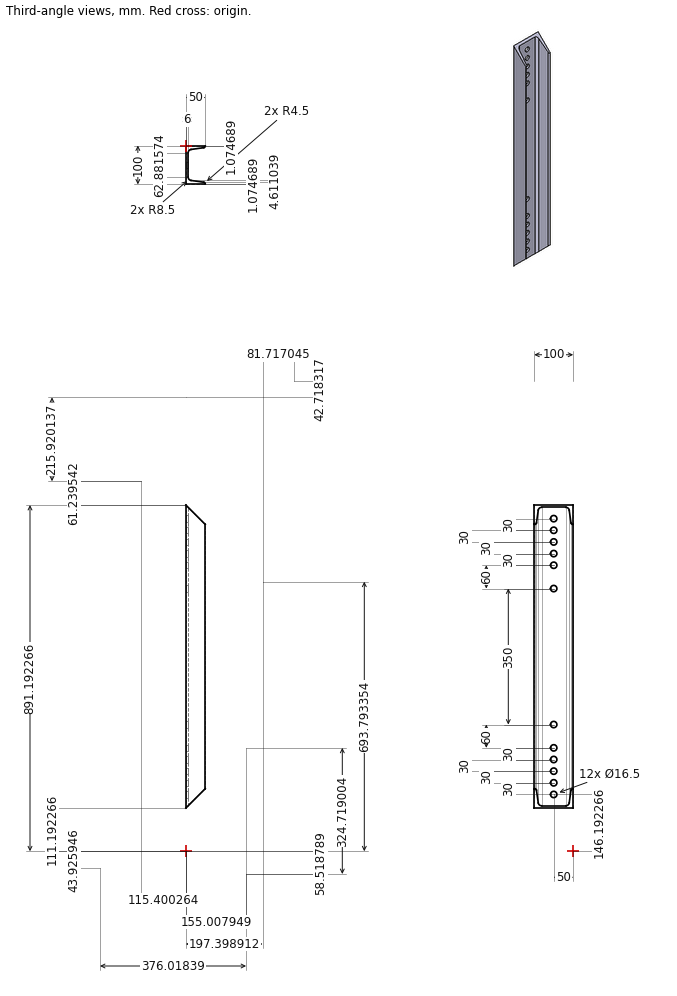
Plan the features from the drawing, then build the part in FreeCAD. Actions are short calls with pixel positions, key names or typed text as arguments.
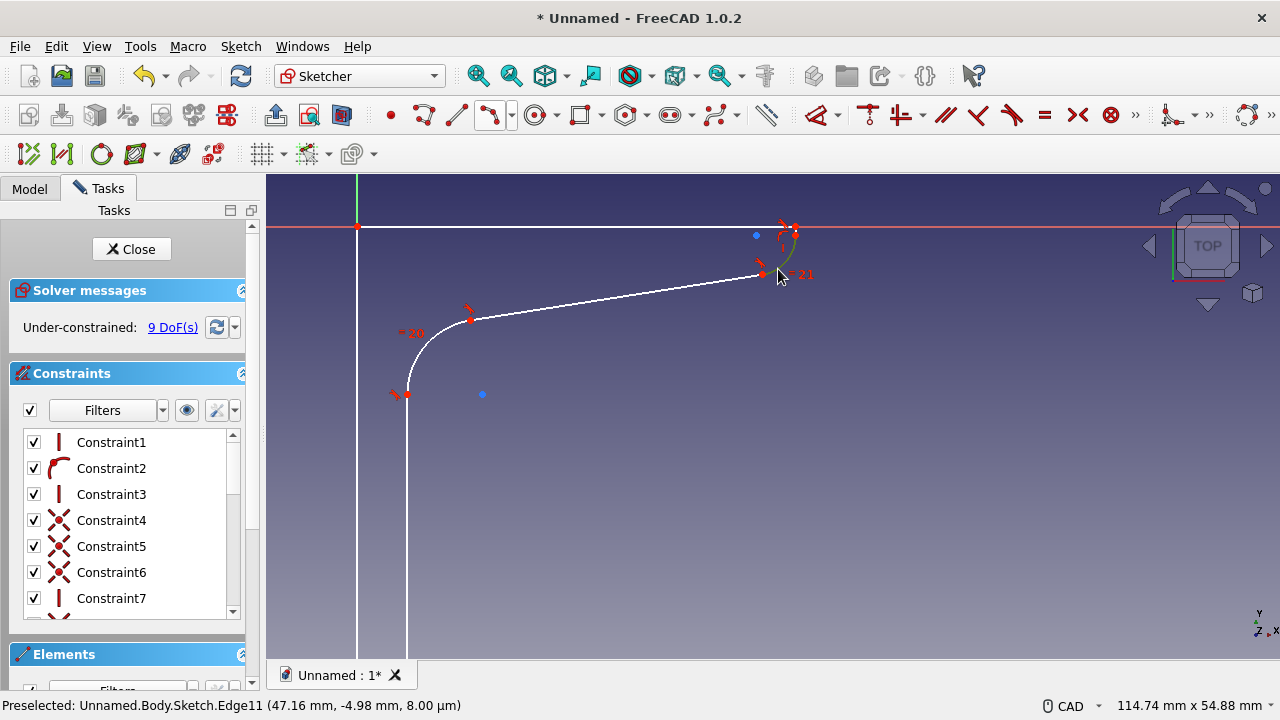
click(838, 116)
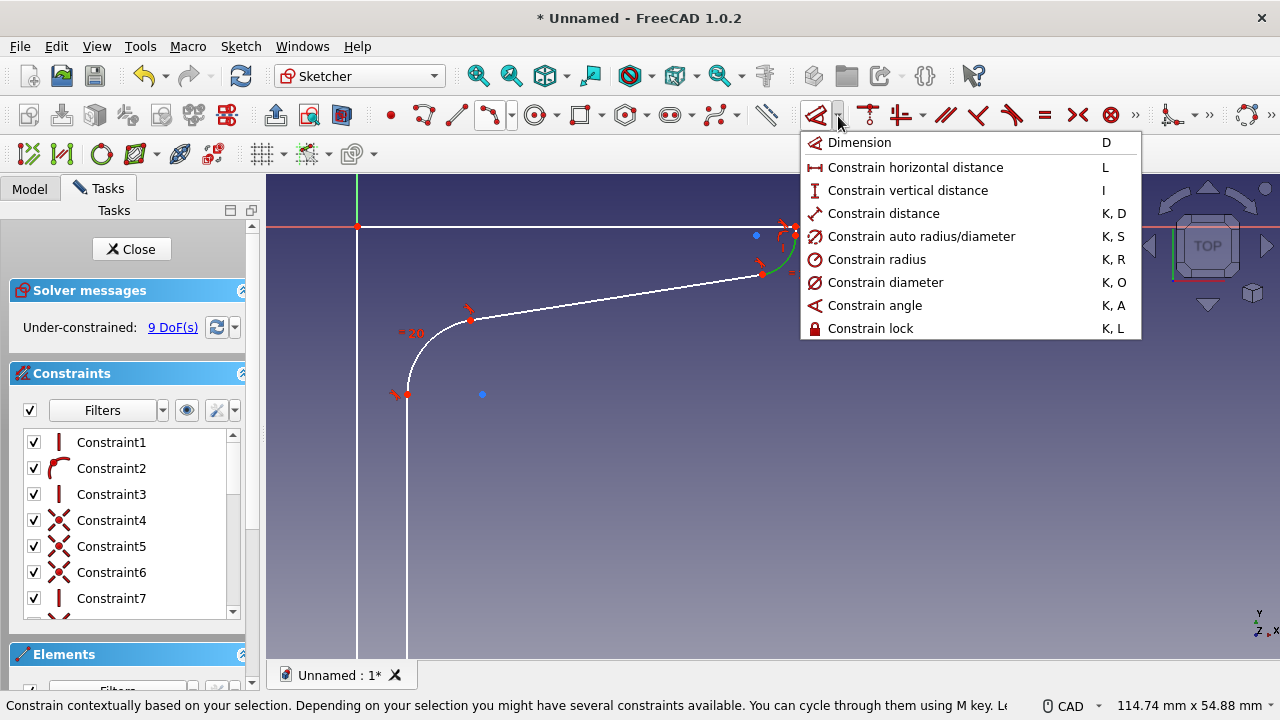
click(971, 260)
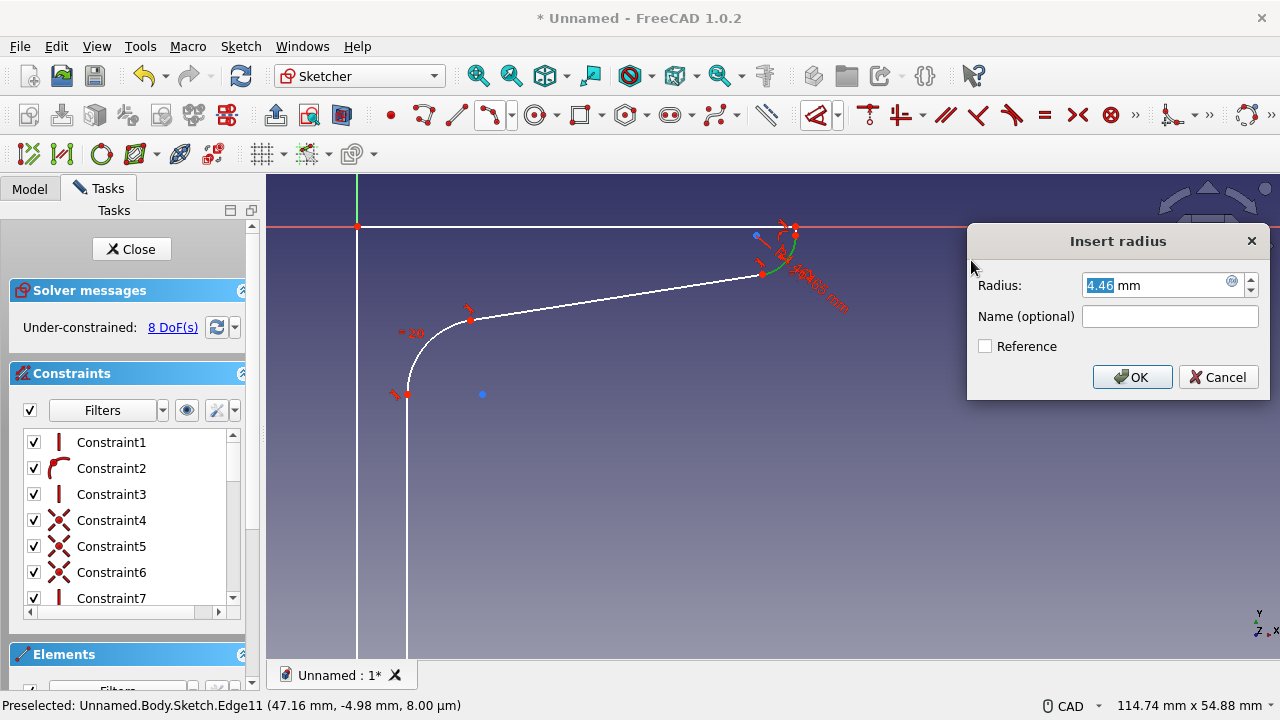
text(4.5)
key(Return)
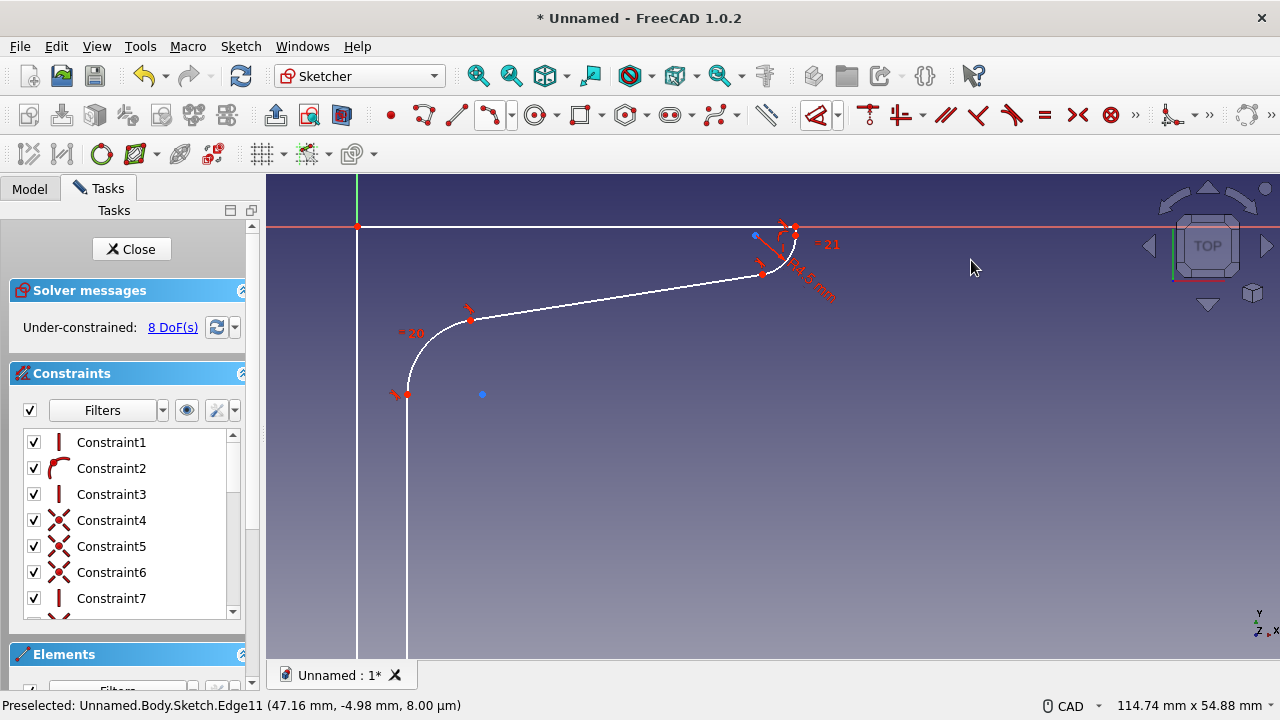
click(664, 227)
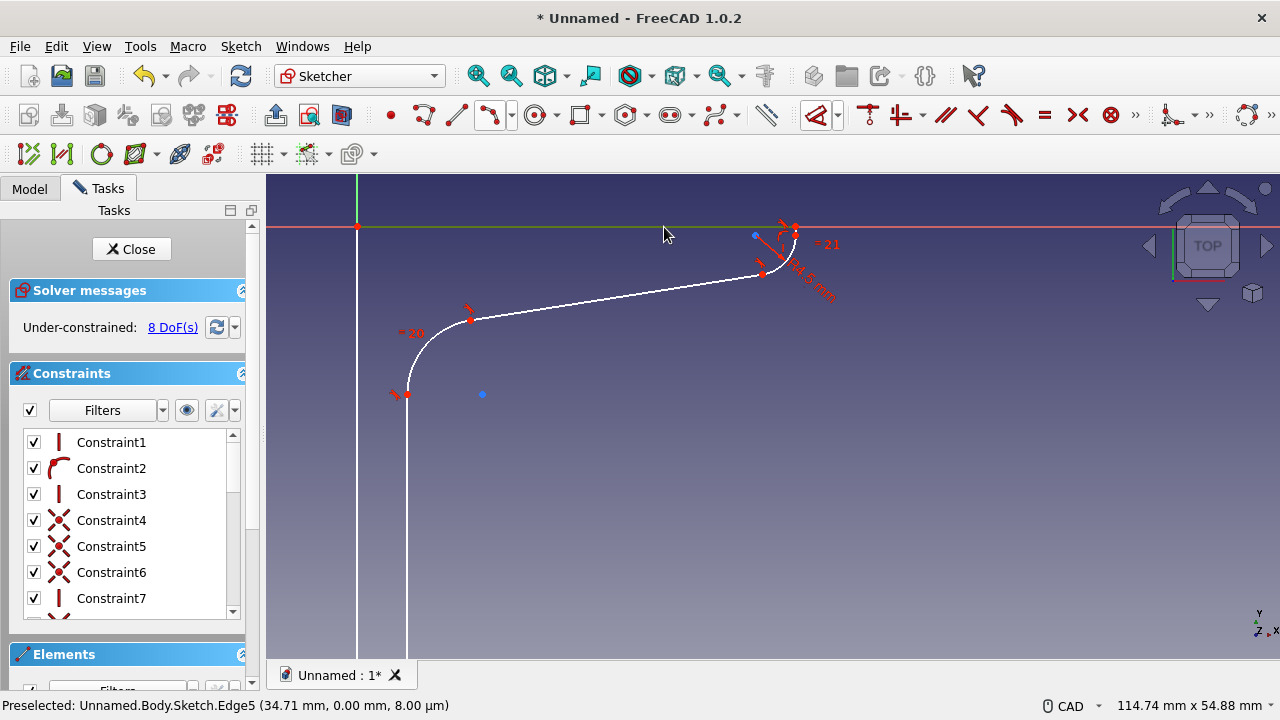
key(l)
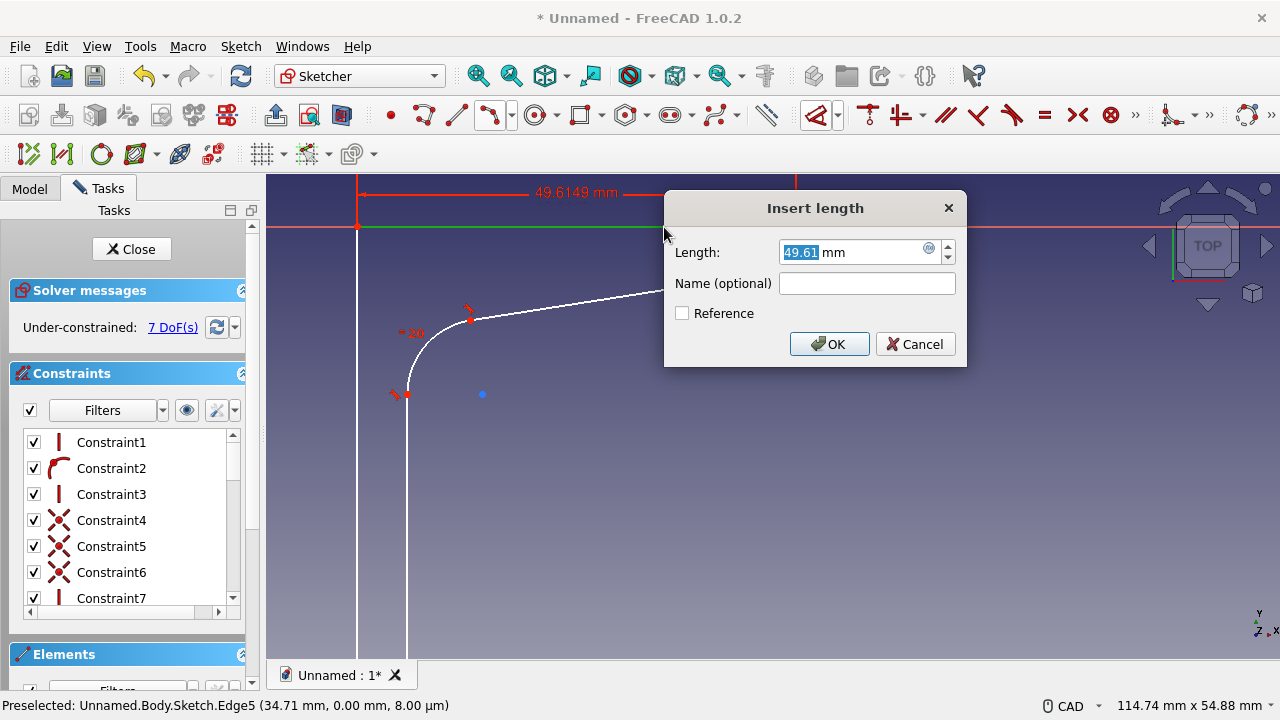
text(50)
key(Return)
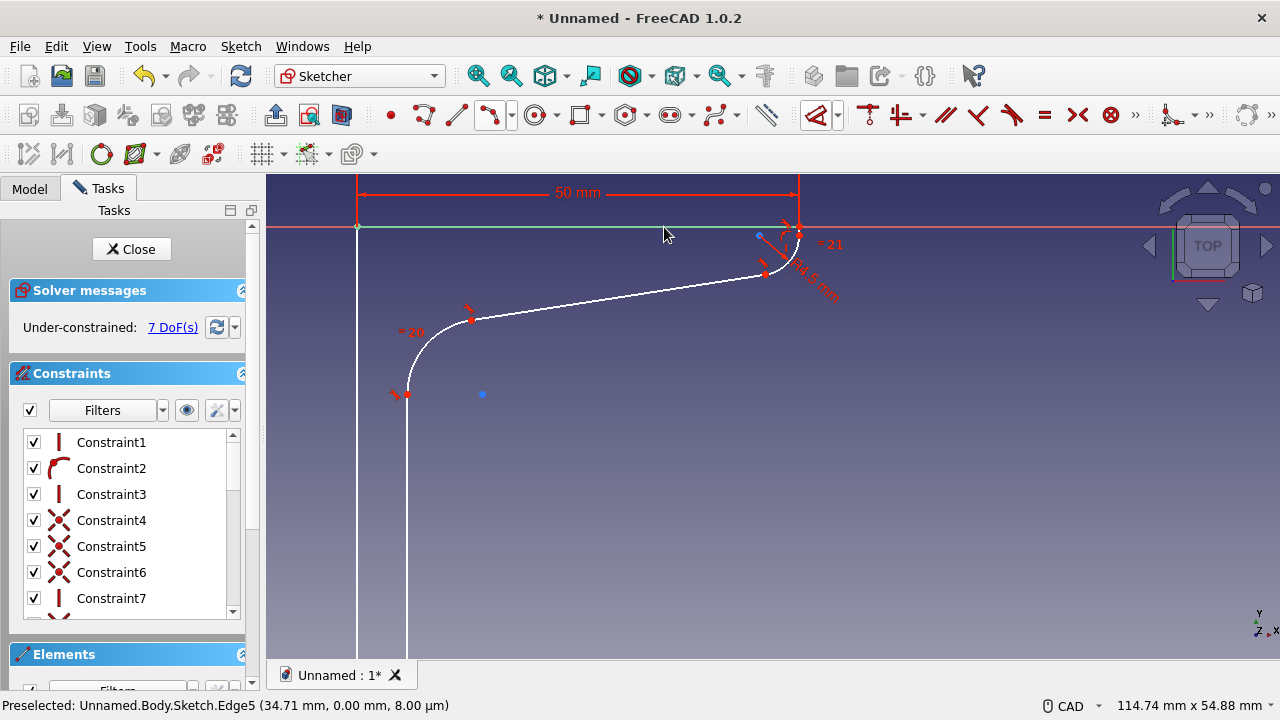
scroll(778, 270, down, 5)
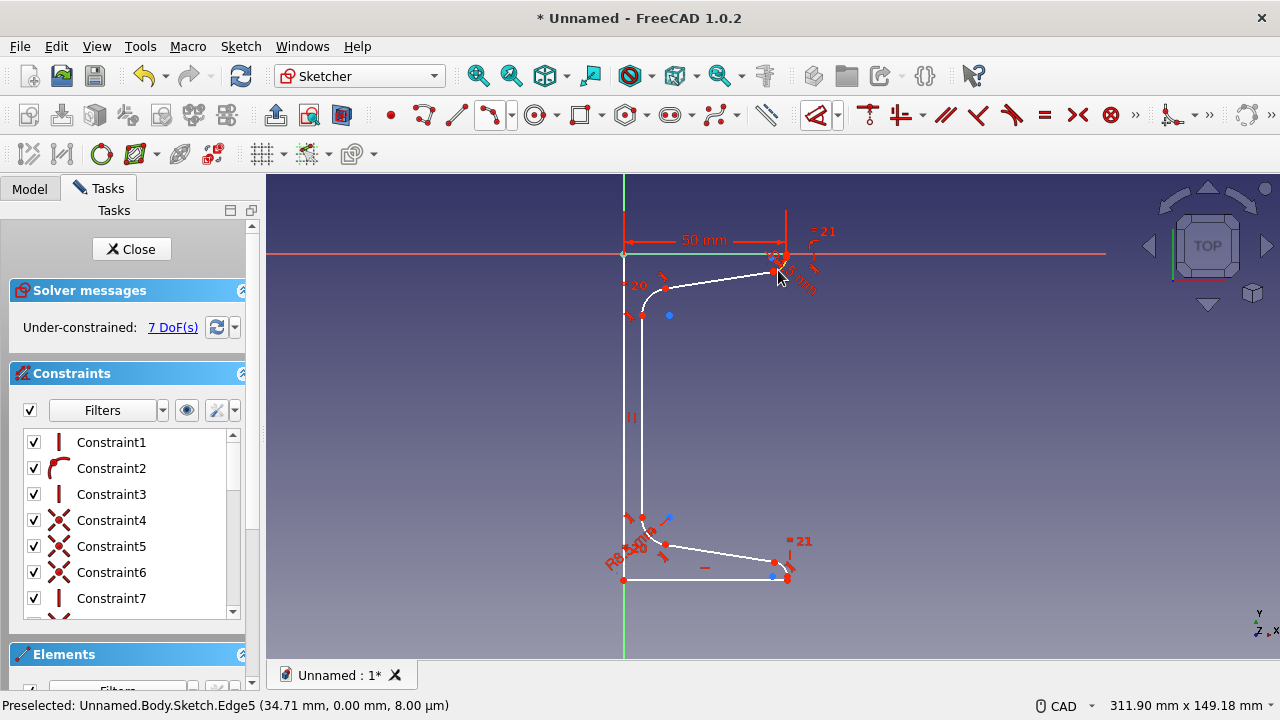
click(673, 580)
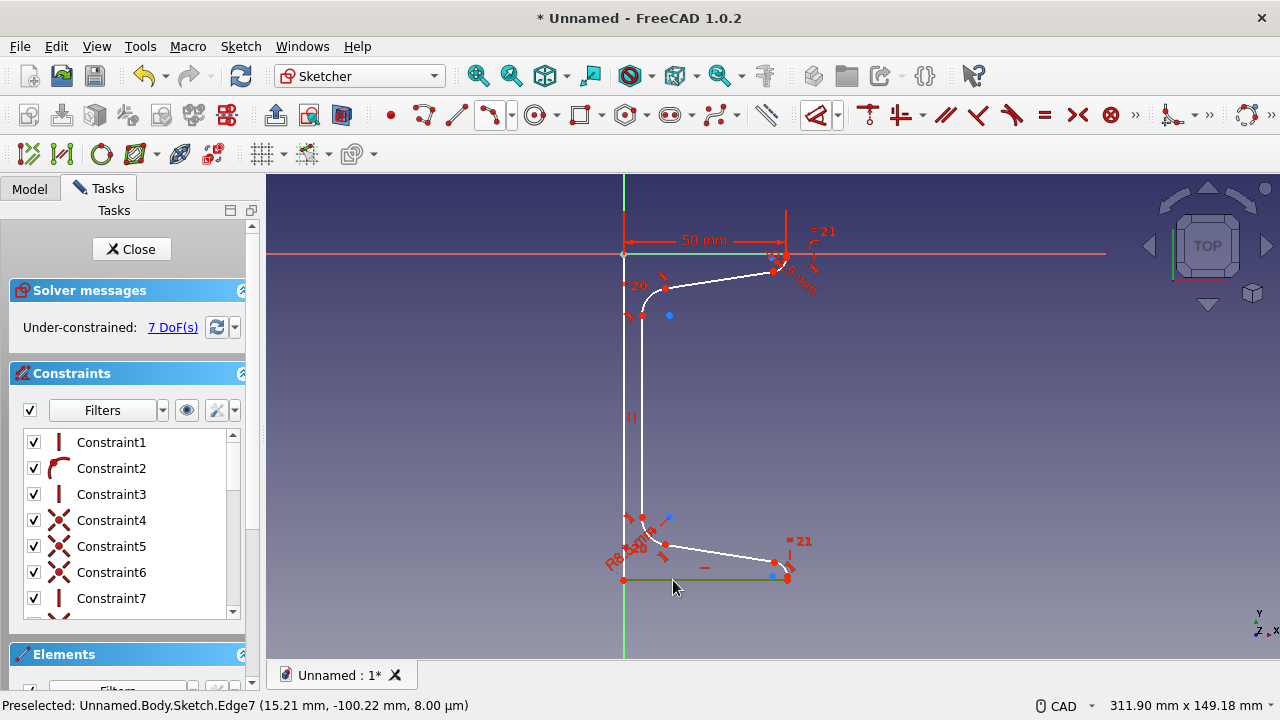
click(838, 116)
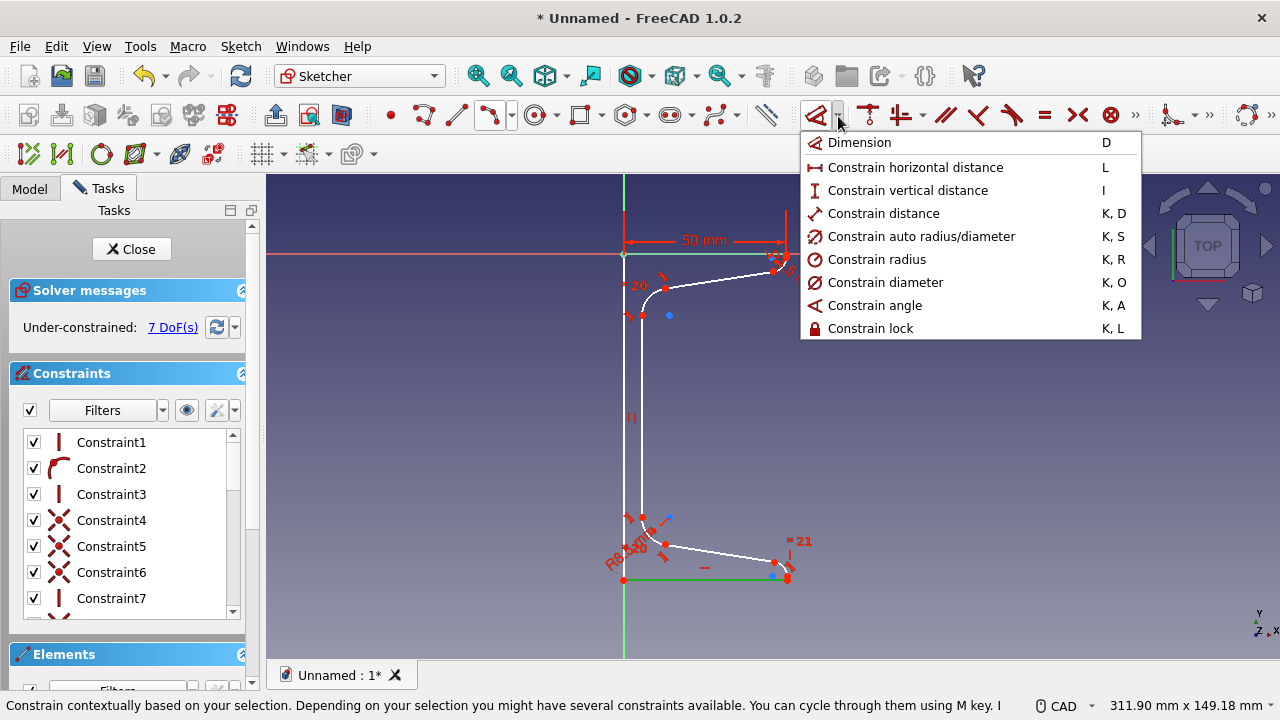
click(971, 168)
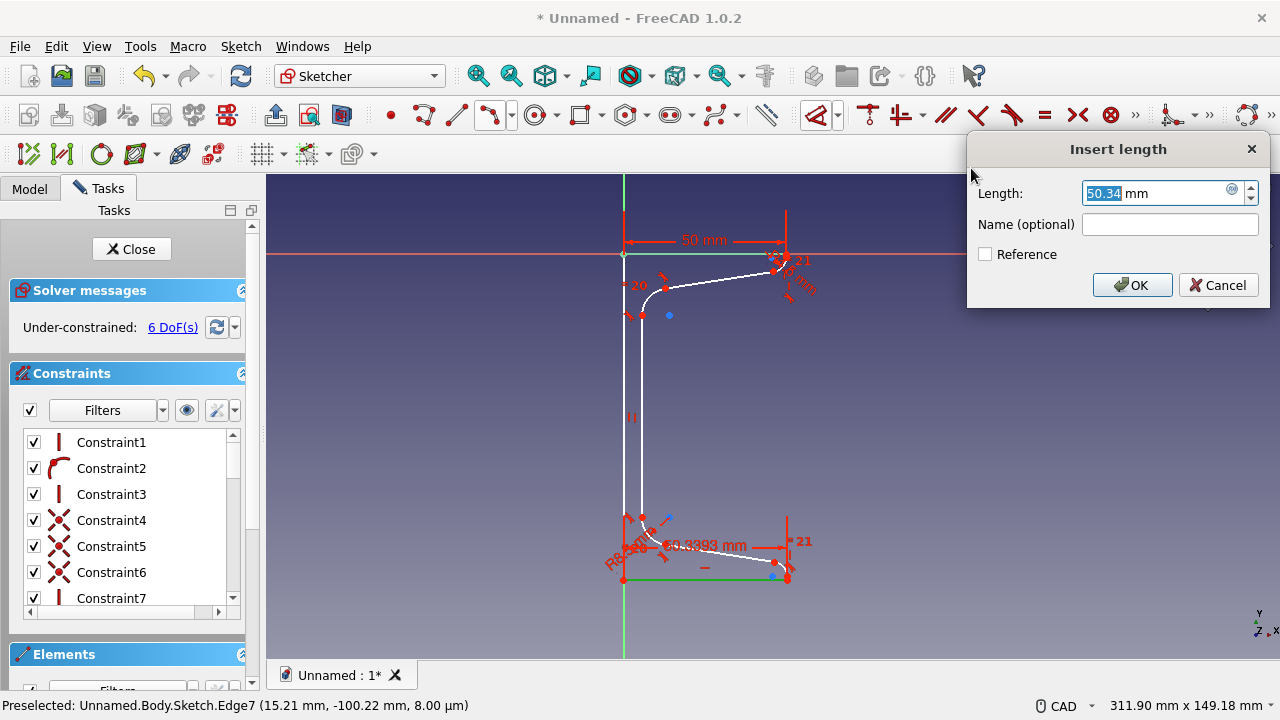
text(50)
key(Return)